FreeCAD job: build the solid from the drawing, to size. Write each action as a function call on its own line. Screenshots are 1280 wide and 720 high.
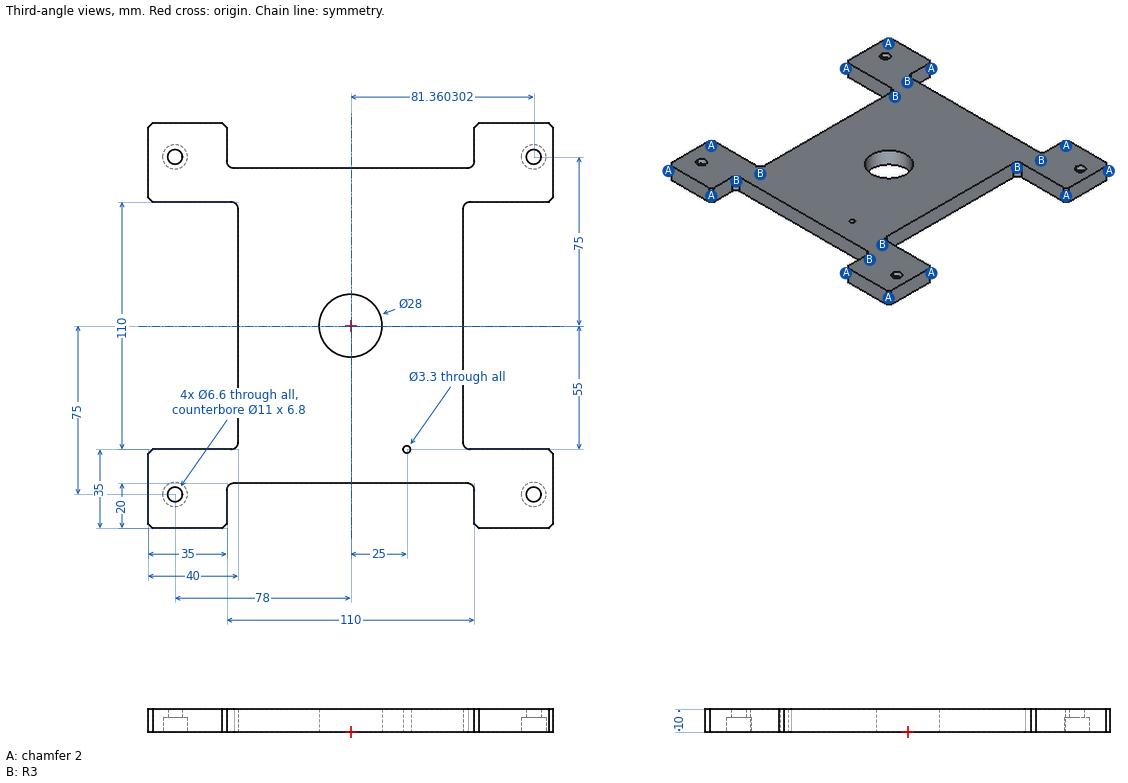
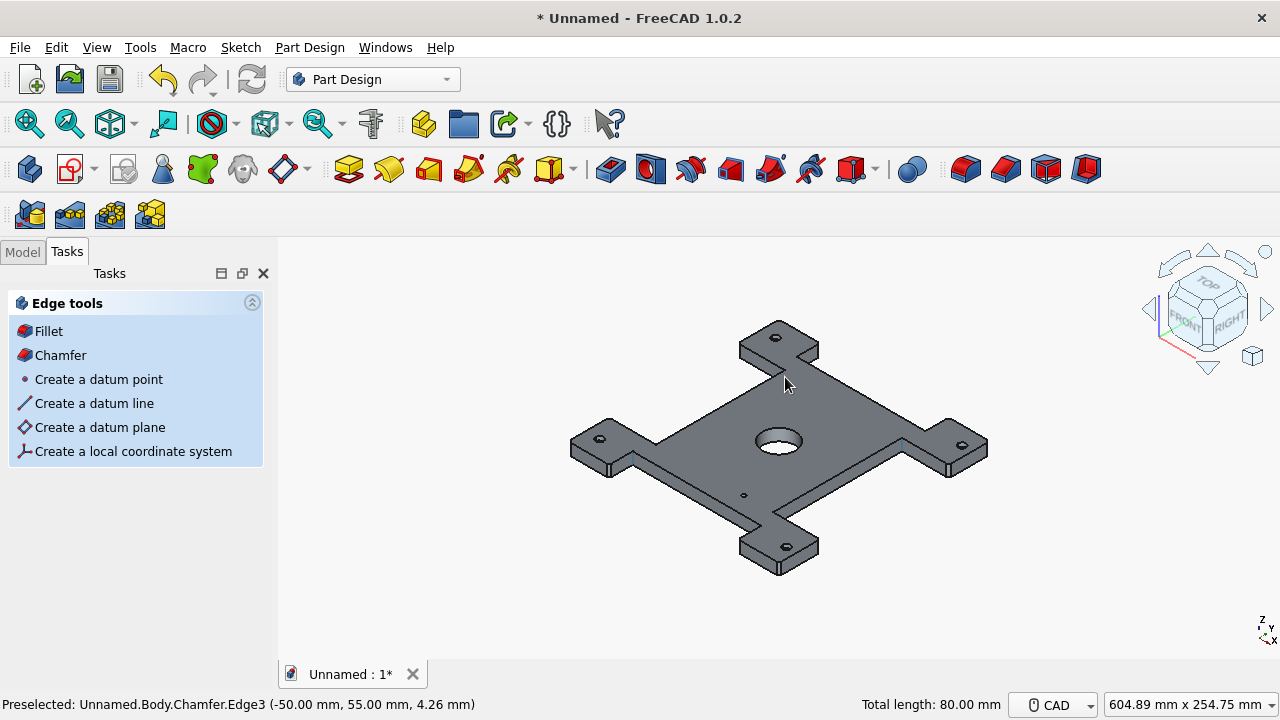
click(966, 170)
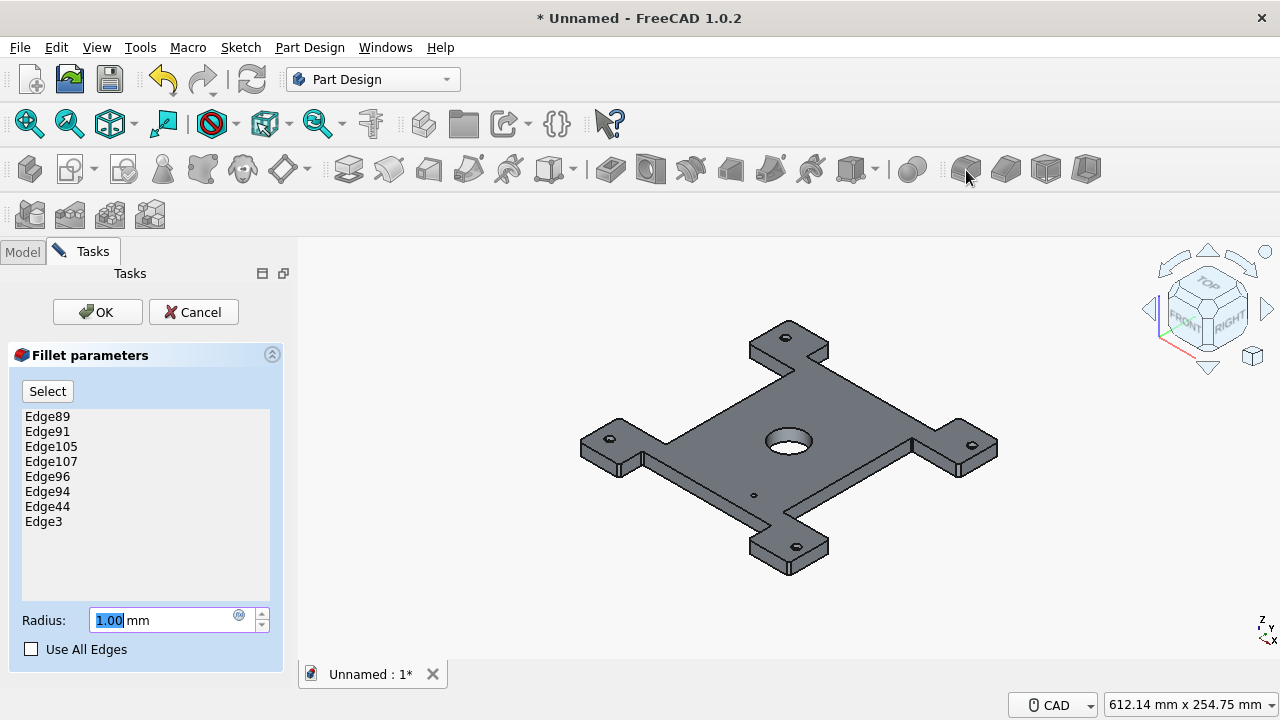
text(3)
key(Tab)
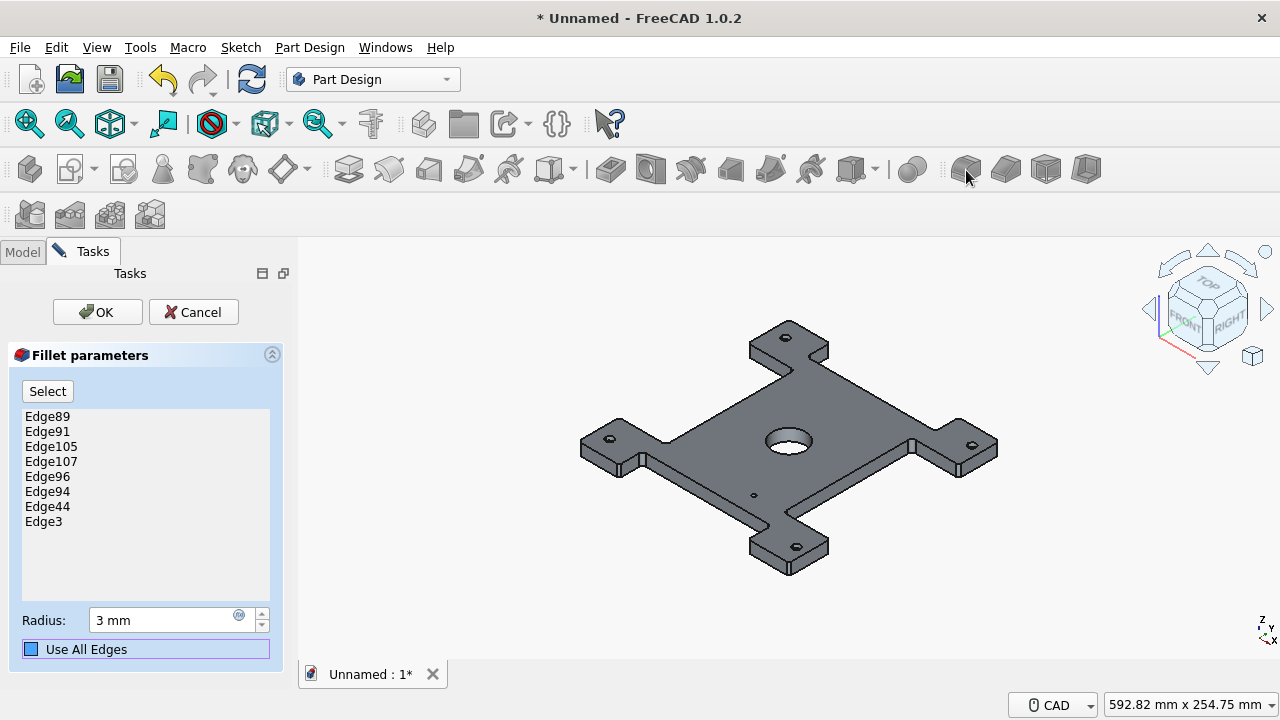
click(98, 312)